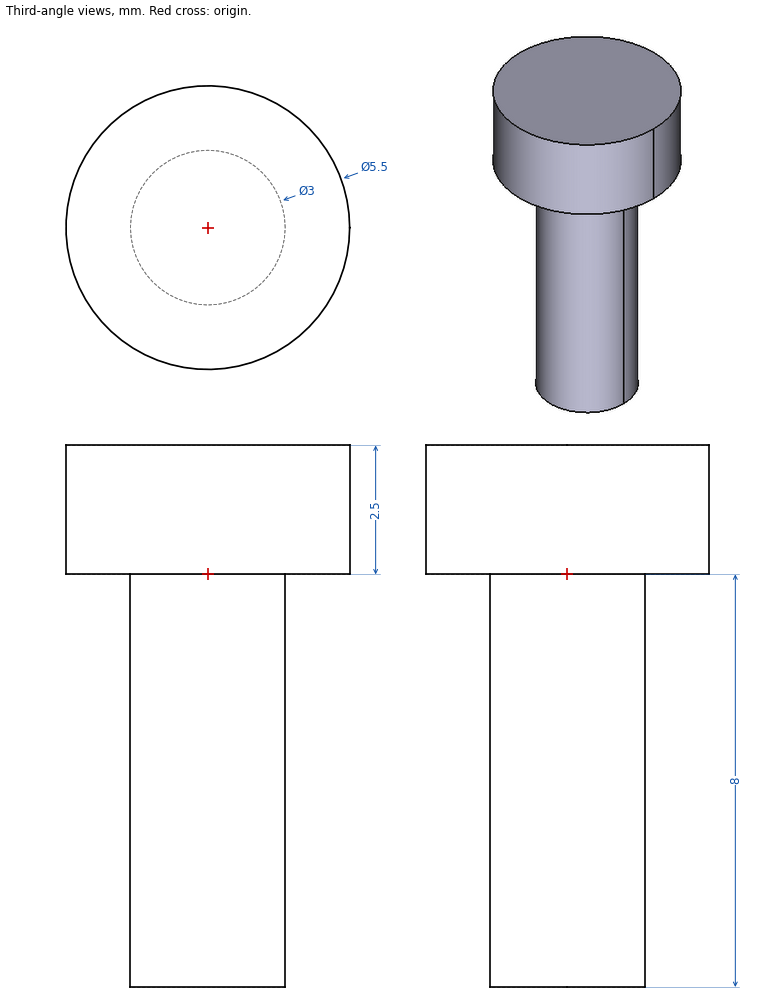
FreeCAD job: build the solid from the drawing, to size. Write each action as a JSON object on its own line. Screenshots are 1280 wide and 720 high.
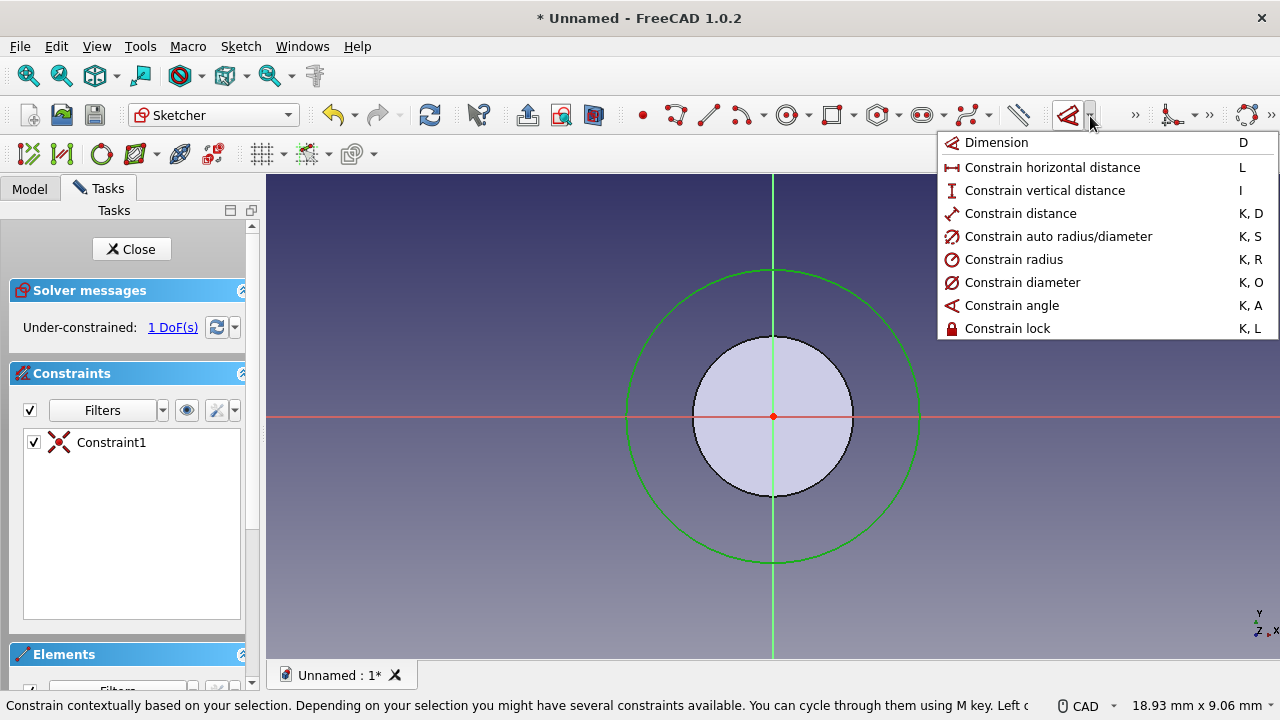
{"action": "left_click", "coordinate": [1108, 282]}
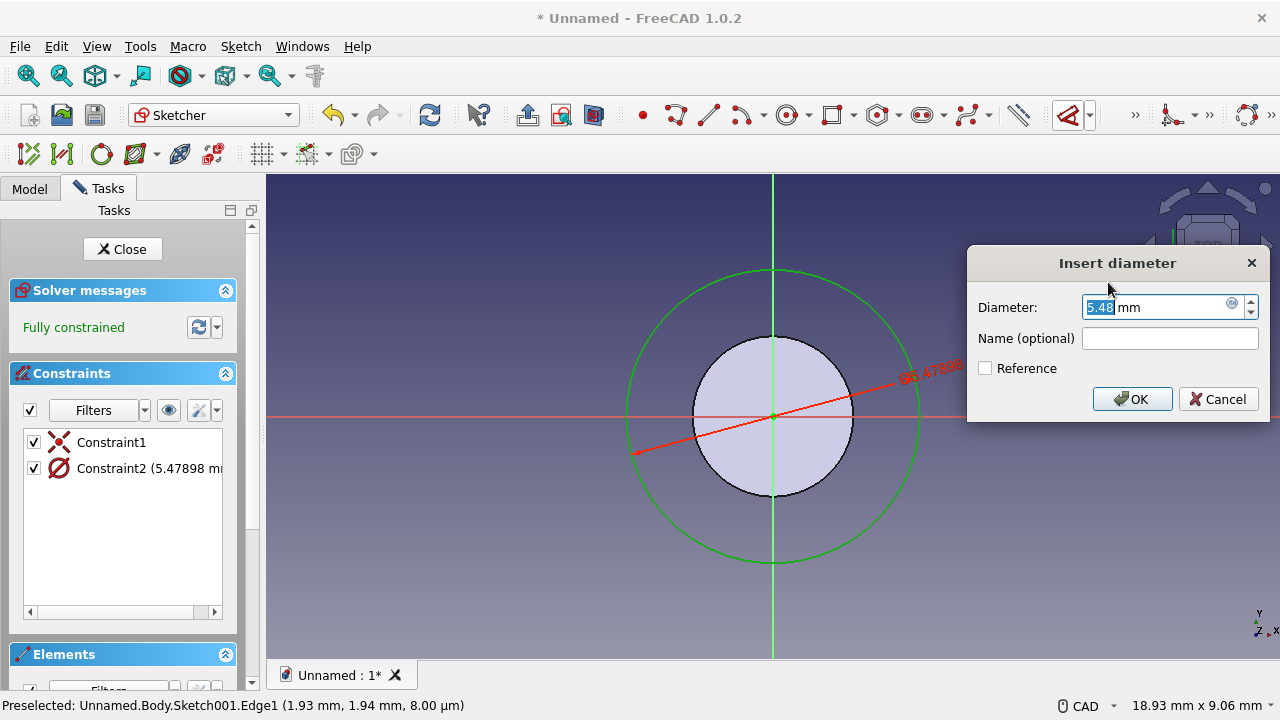
{"action": "type", "text": "5.5"}
{"action": "key", "text": "Return"}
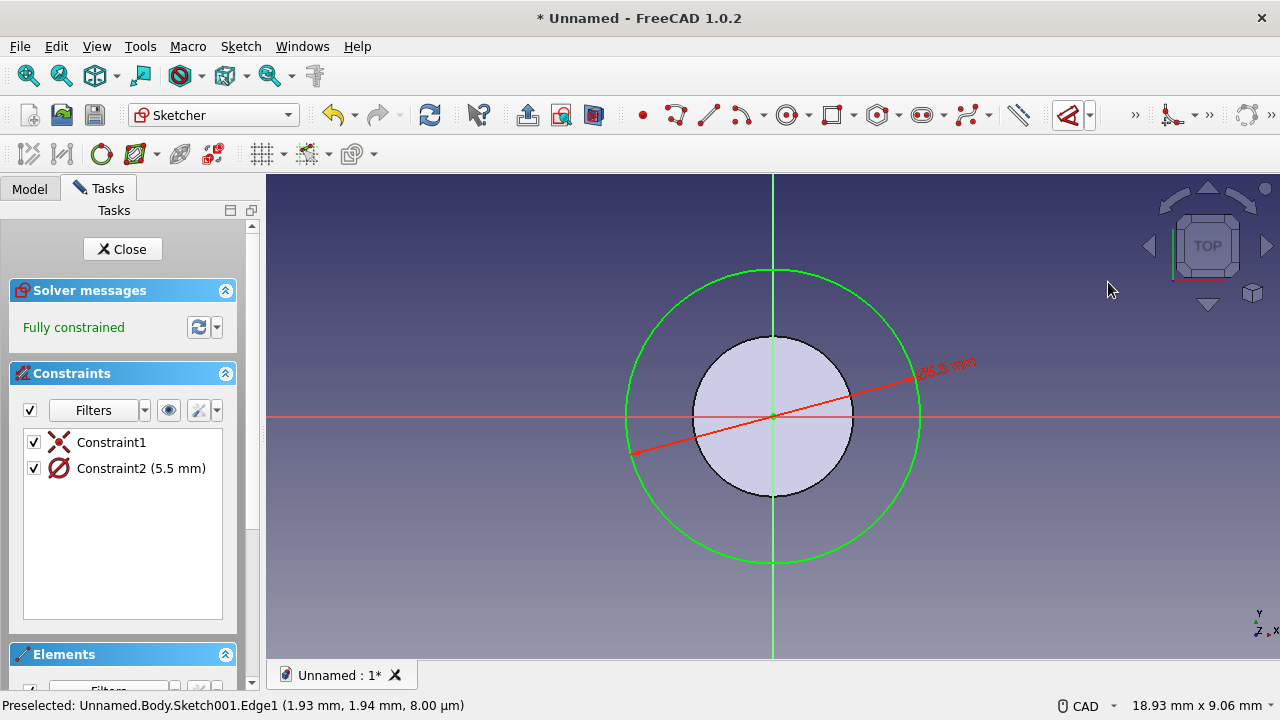
{"action": "left_click", "coordinate": [123, 249]}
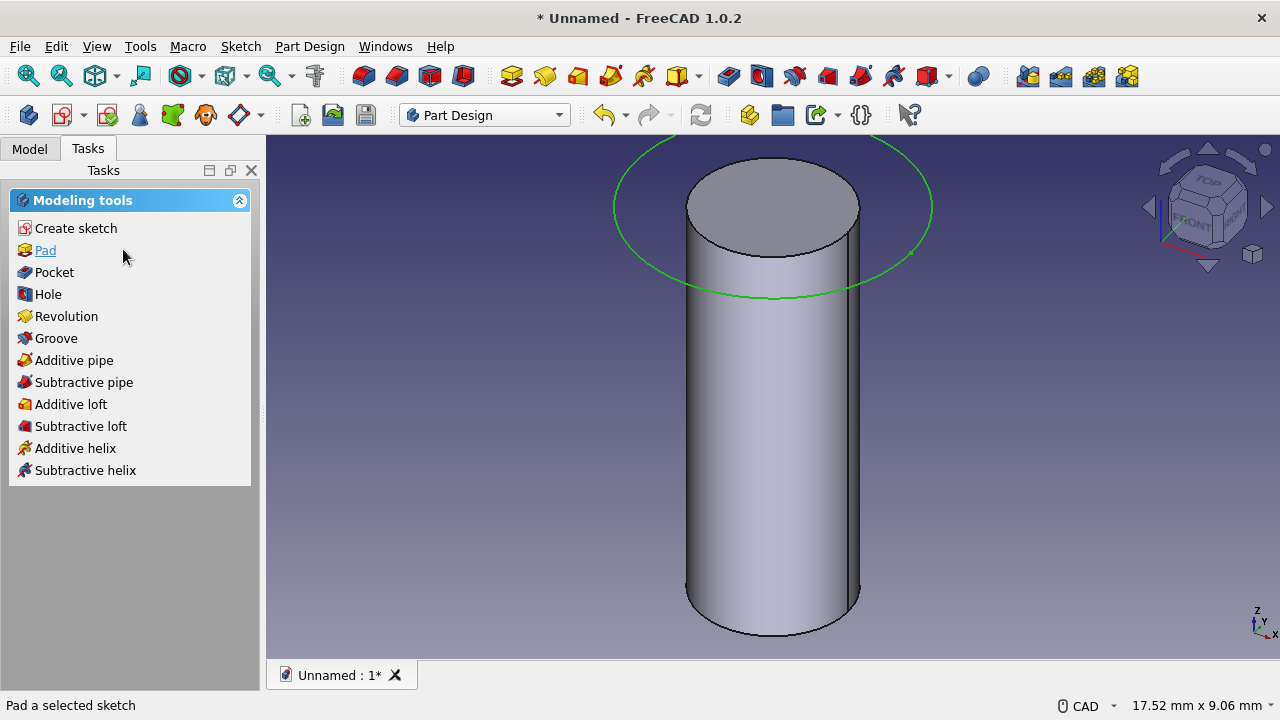
{"action": "left_click", "coordinate": [512, 76]}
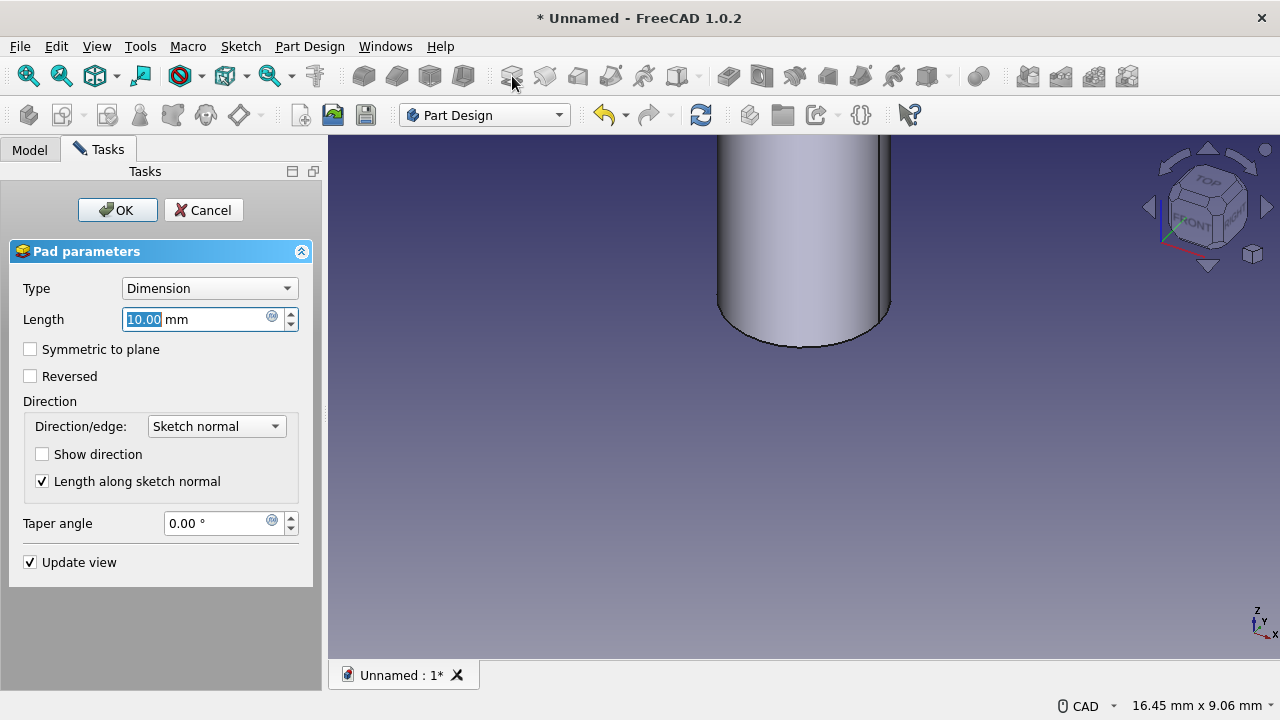
{"action": "type", "text": "2.5"}
{"action": "key", "text": "Tab"}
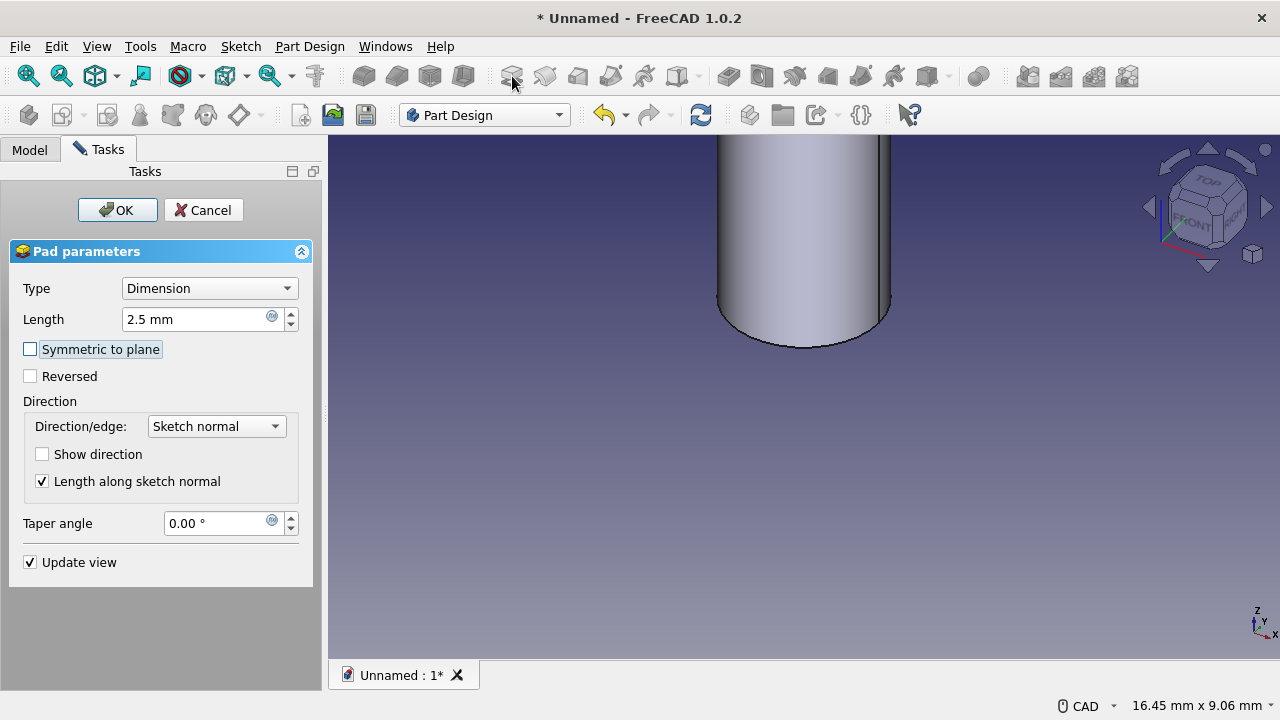
{"action": "left_click", "coordinate": [118, 210]}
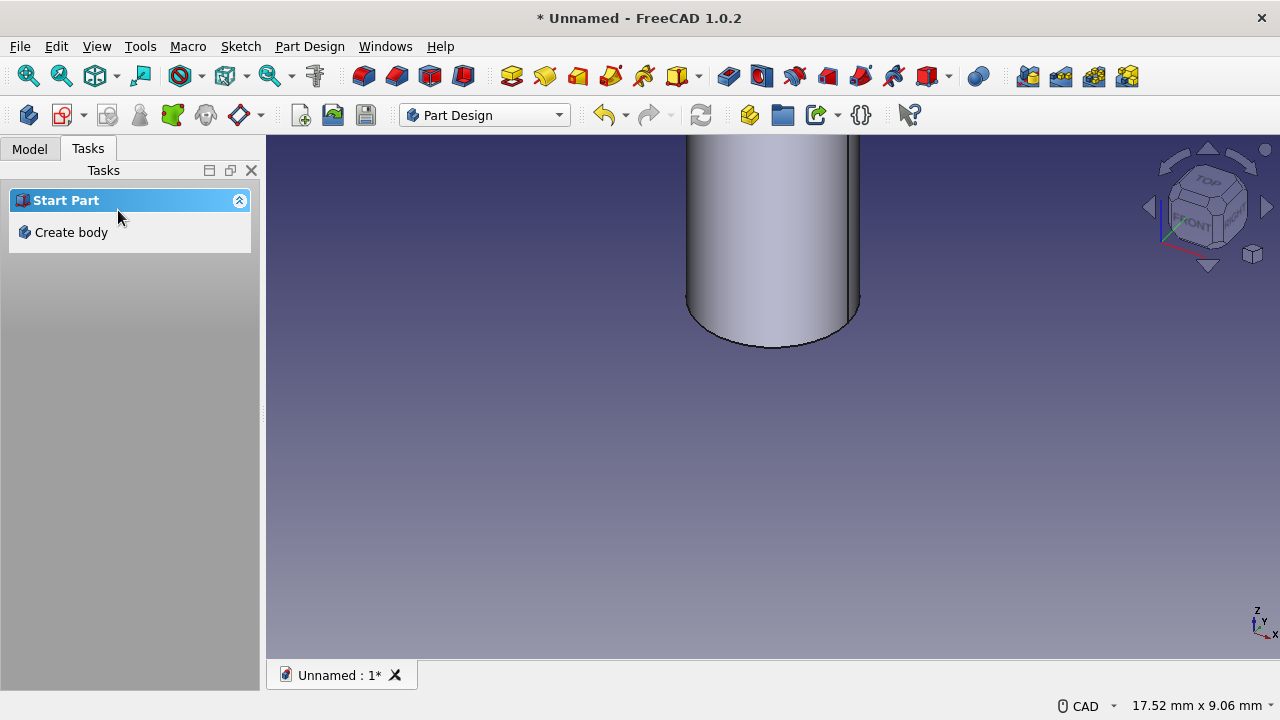
{"action": "key", "text": "0"}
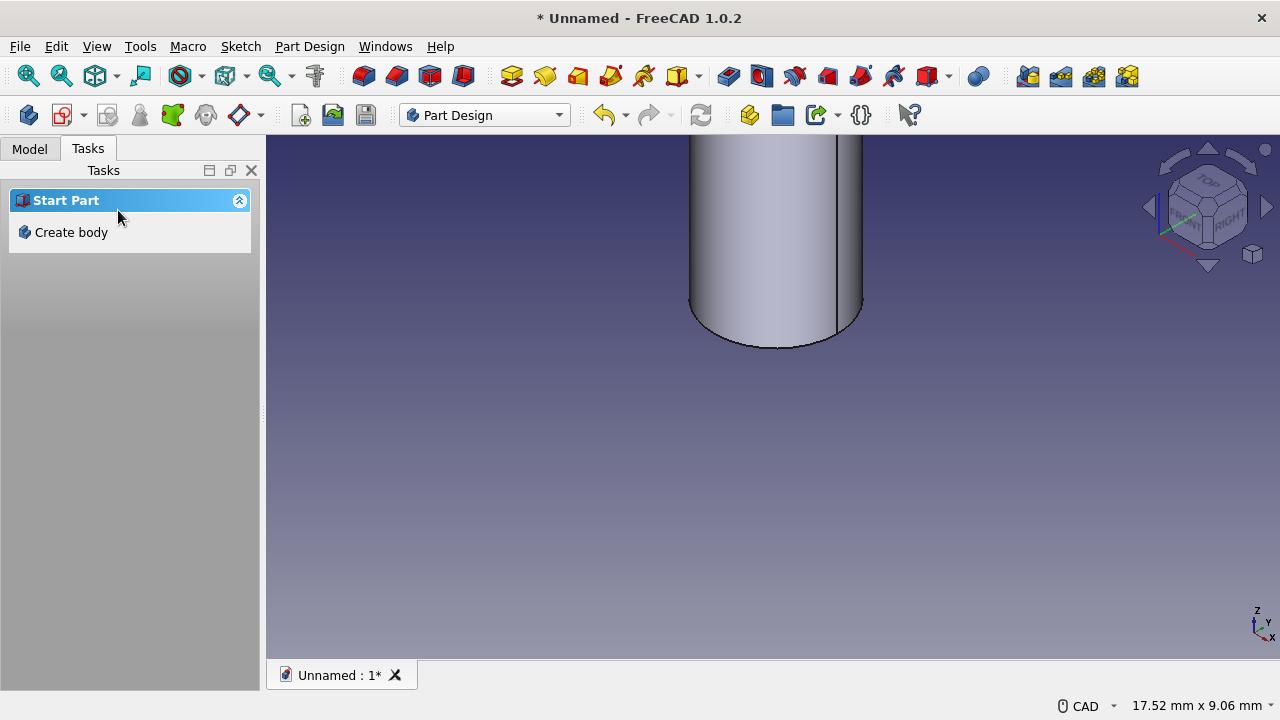
{"action": "left_click", "coordinate": [29, 76]}